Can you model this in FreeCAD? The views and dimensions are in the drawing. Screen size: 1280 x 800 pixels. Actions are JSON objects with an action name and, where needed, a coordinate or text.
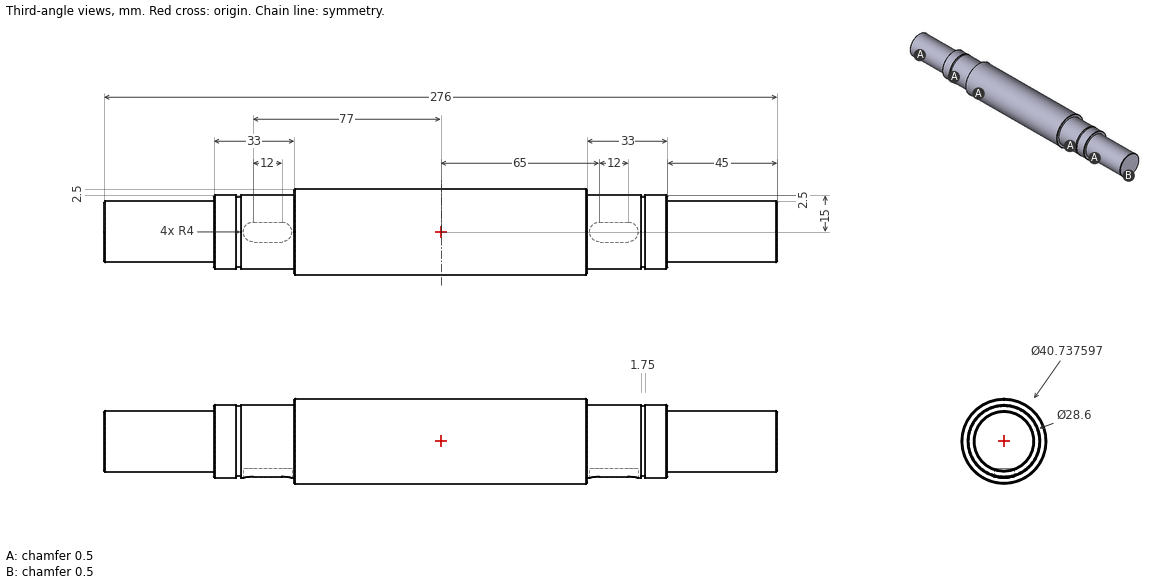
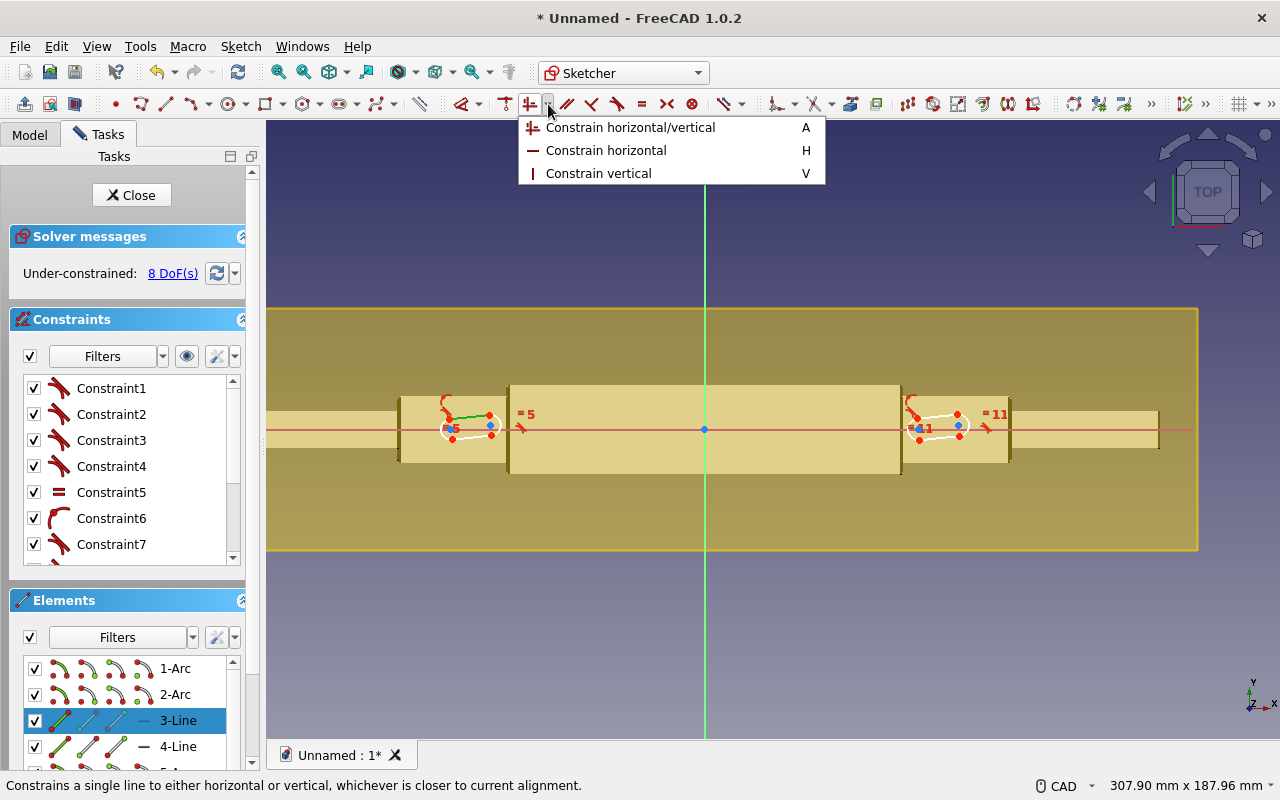
{"action": "left_click", "coordinate": [672, 150]}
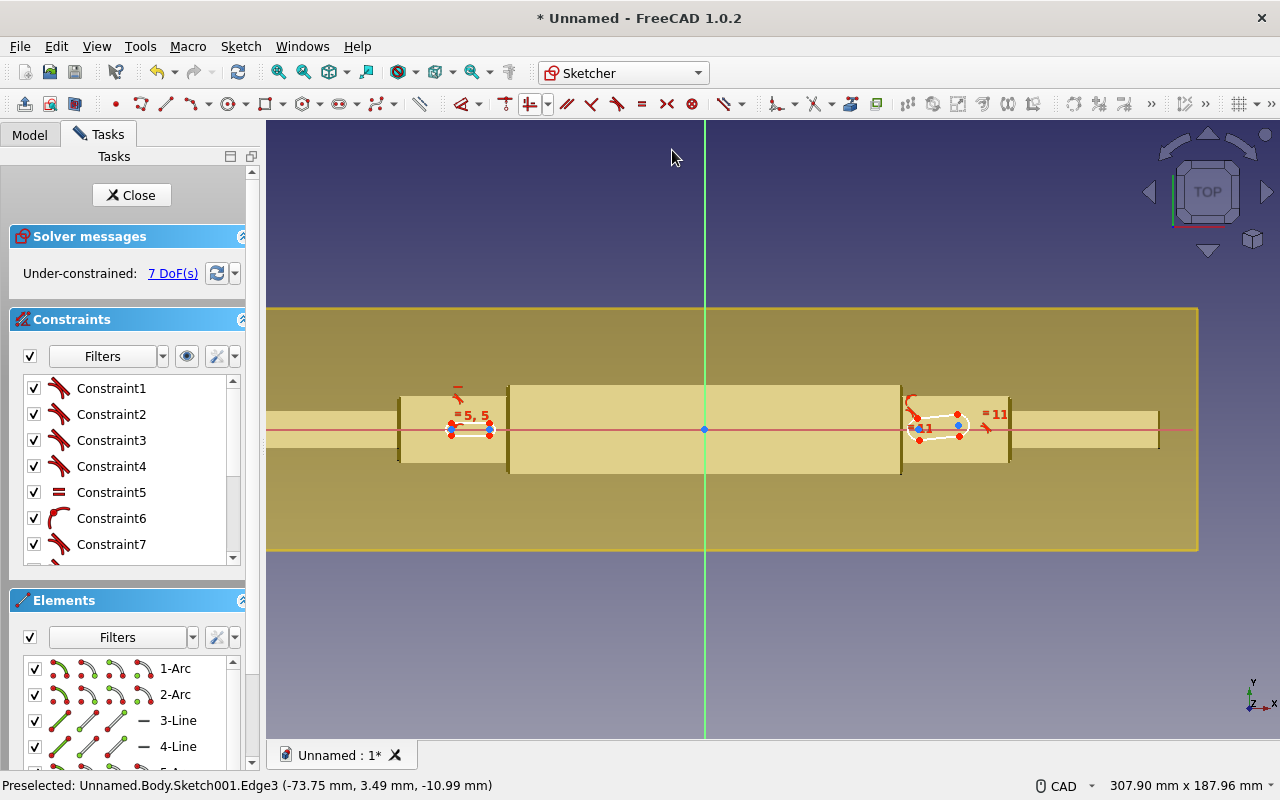
{"action": "left_click", "coordinate": [945, 416]}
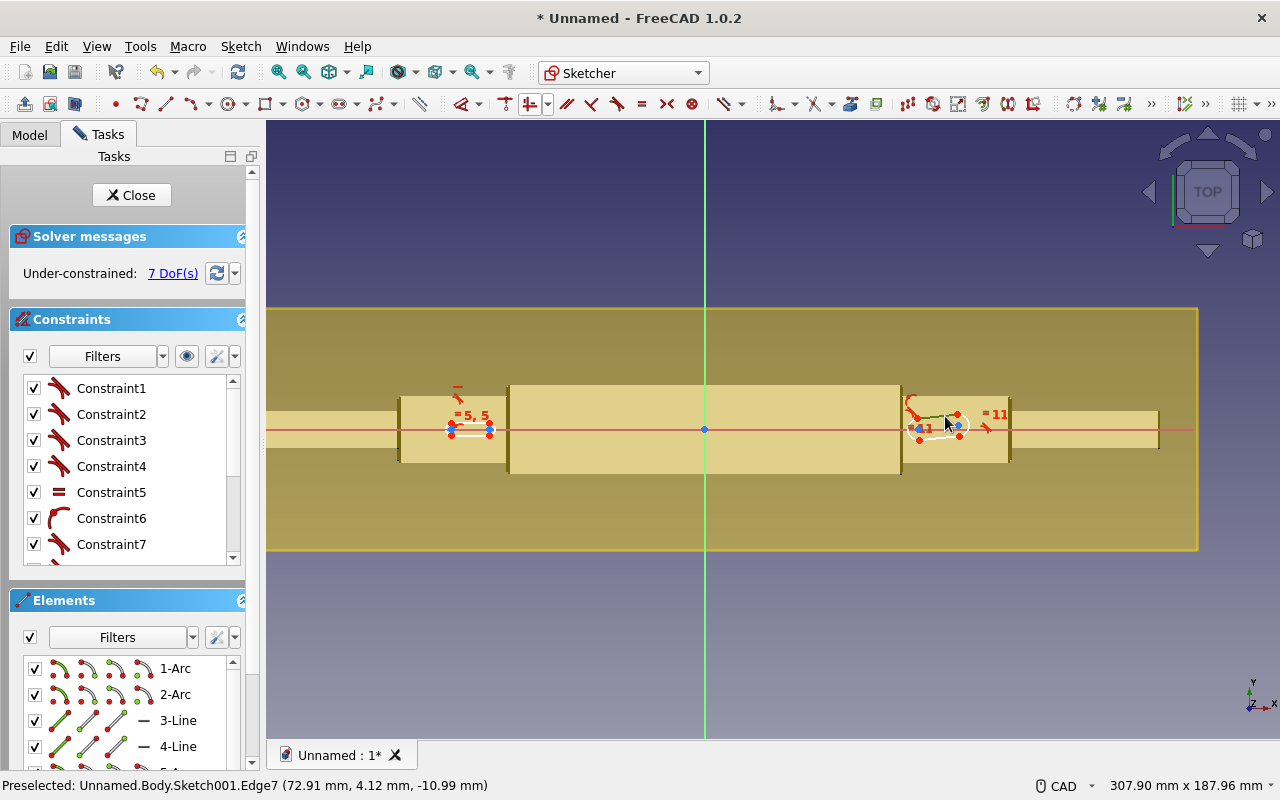
{"action": "key", "text": "h"}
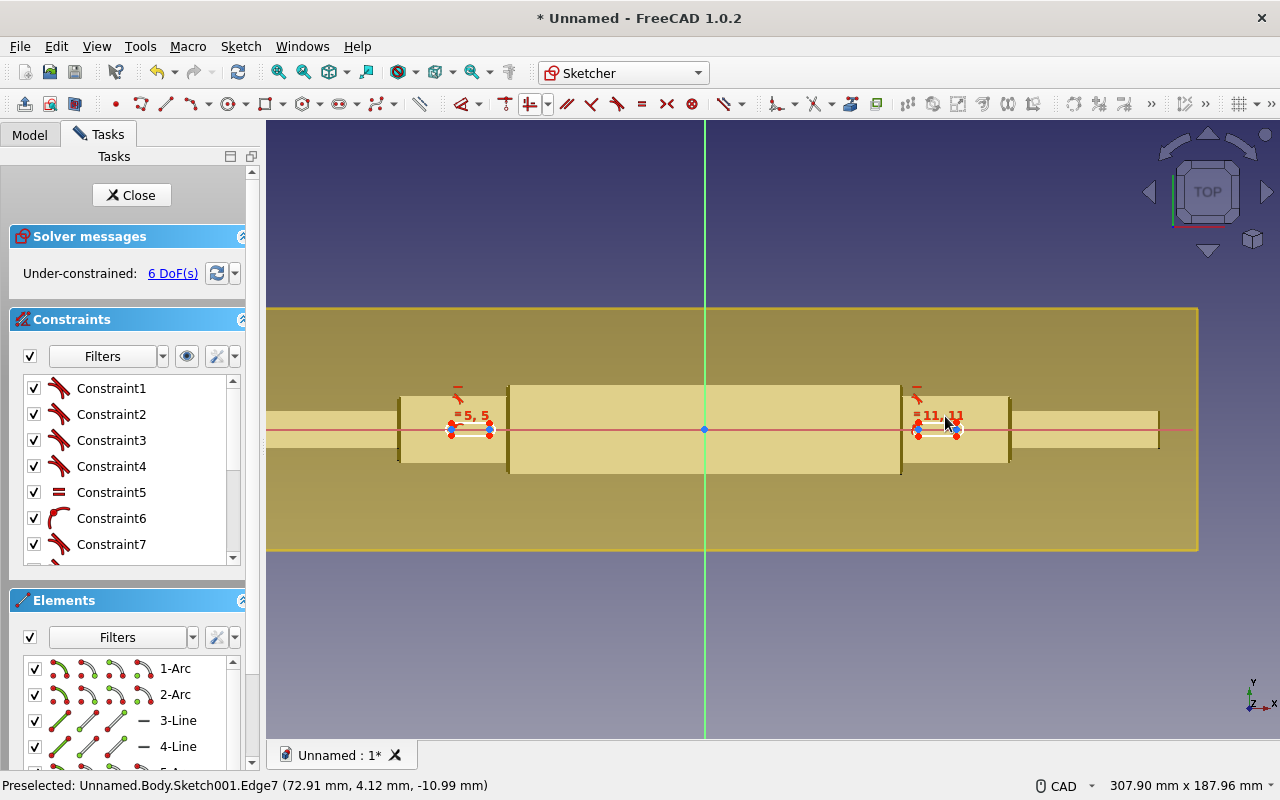
{"action": "scroll", "coordinate": [446, 430], "scroll_direction": "up", "scroll_amount": 5}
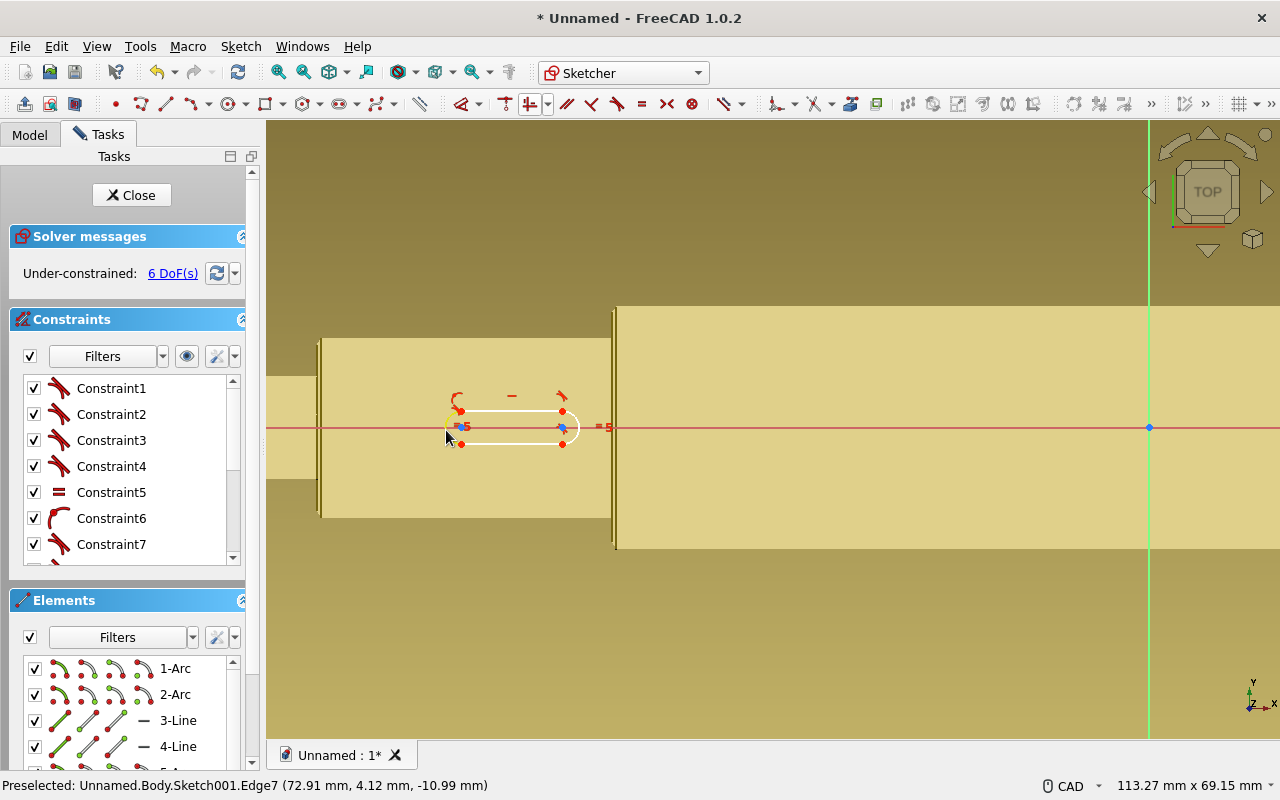
{"action": "left_click", "coordinate": [446, 428]}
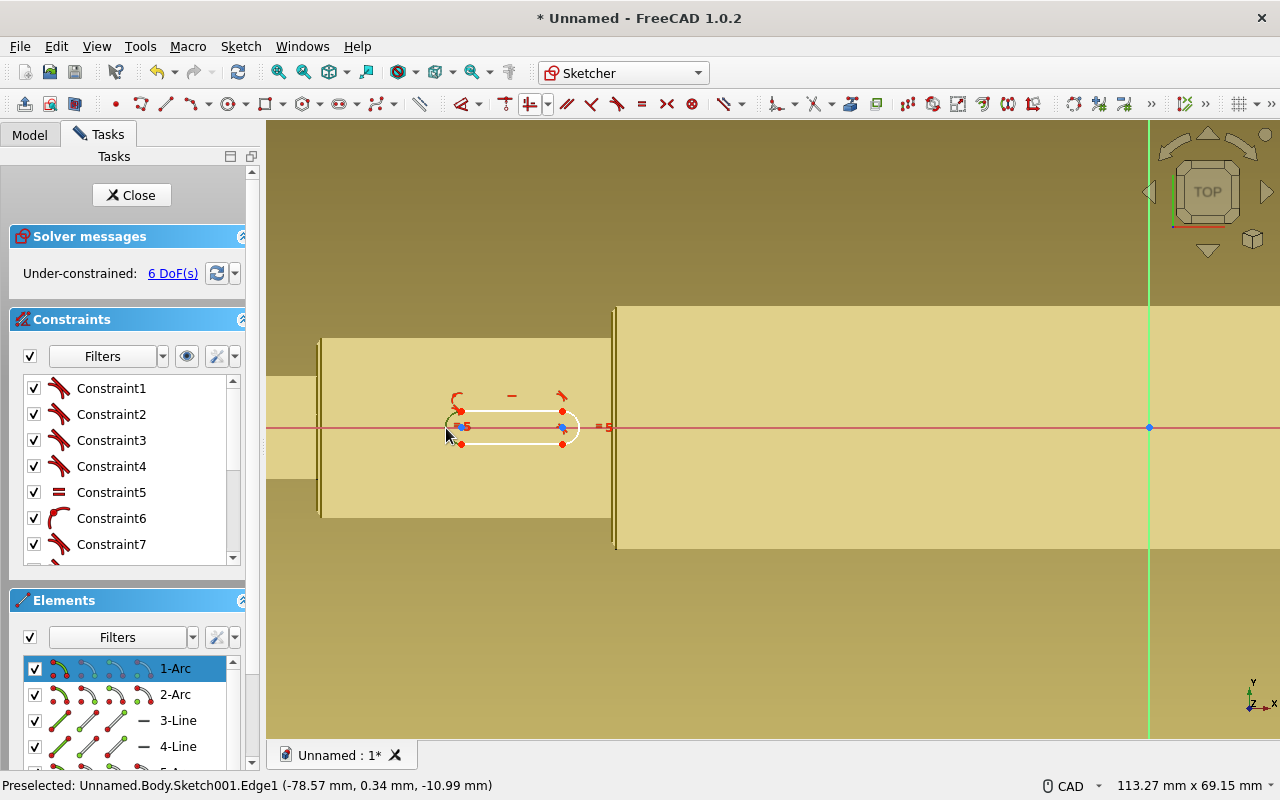
{"action": "scroll", "coordinate": [446, 431], "scroll_direction": "down", "scroll_amount": 5}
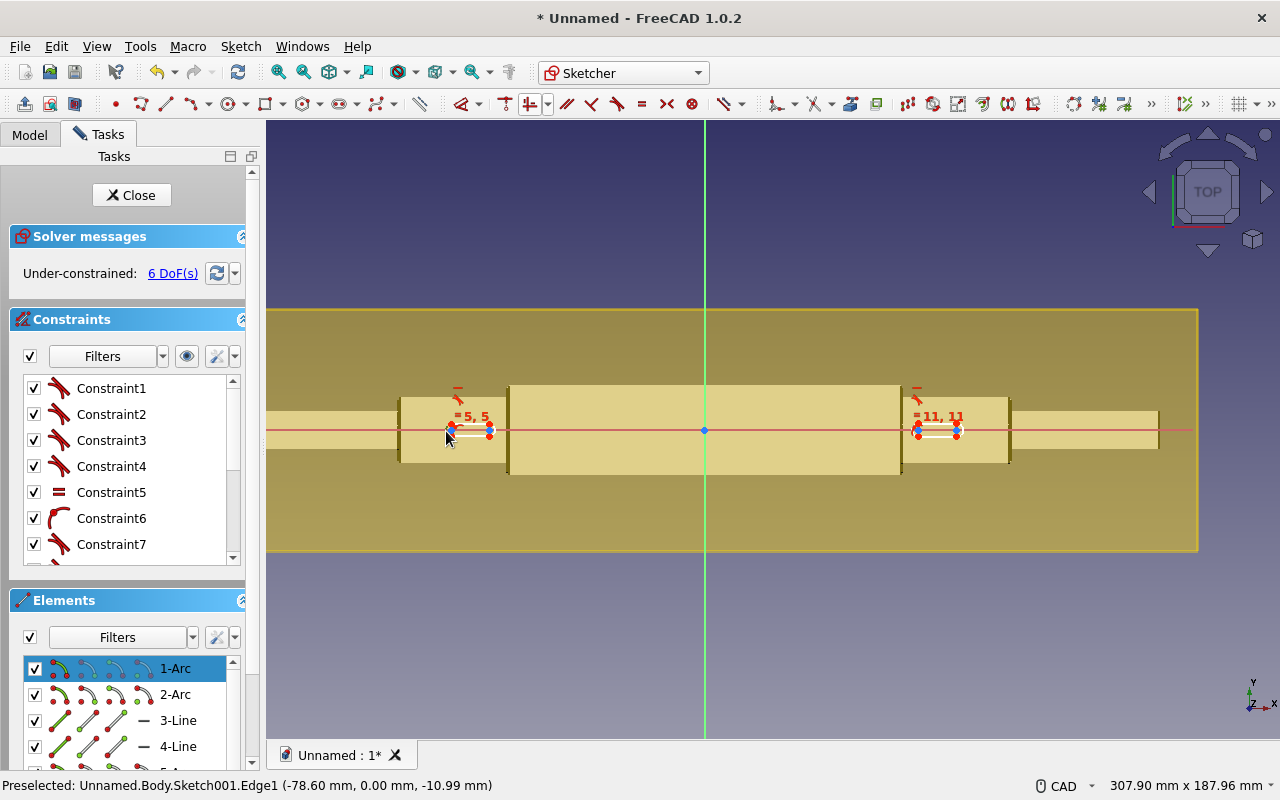
{"action": "scroll", "coordinate": [914, 426], "scroll_direction": "up", "scroll_amount": 7}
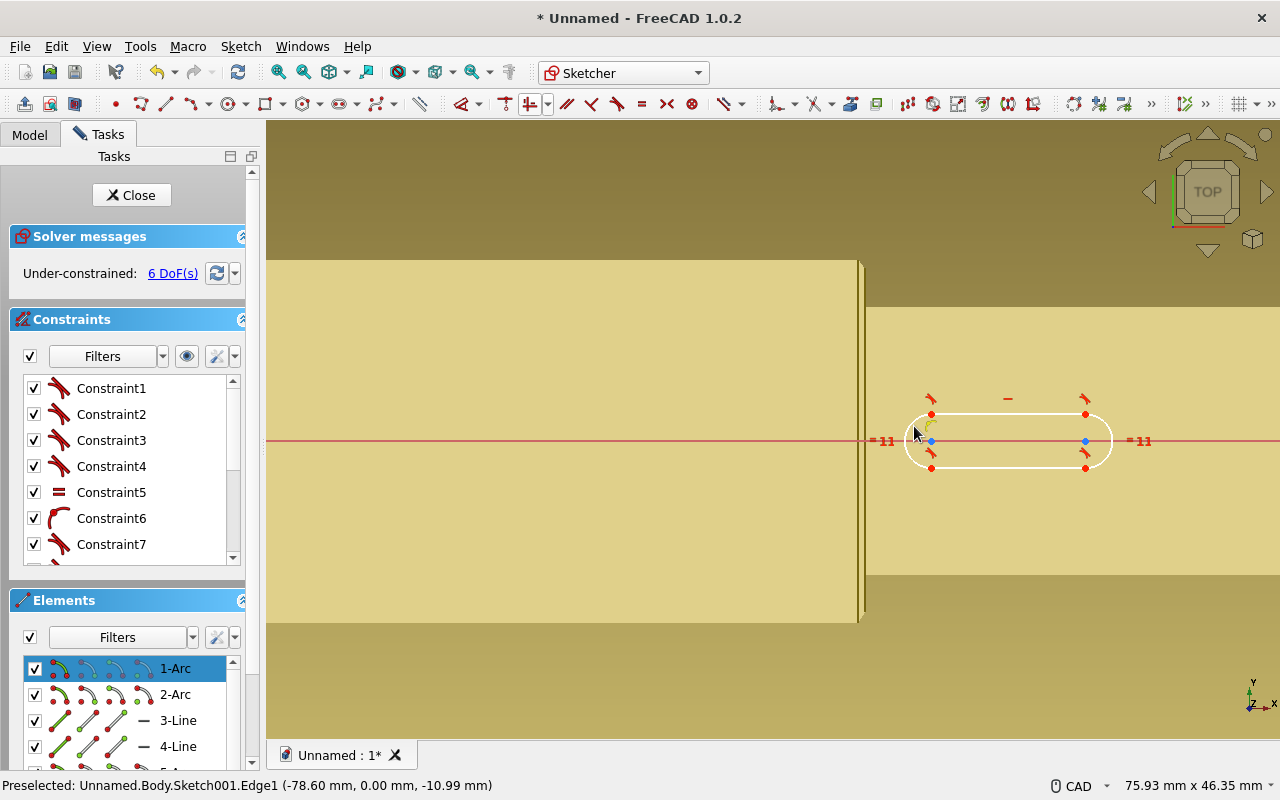
{"action": "left_click", "coordinate": [910, 425]}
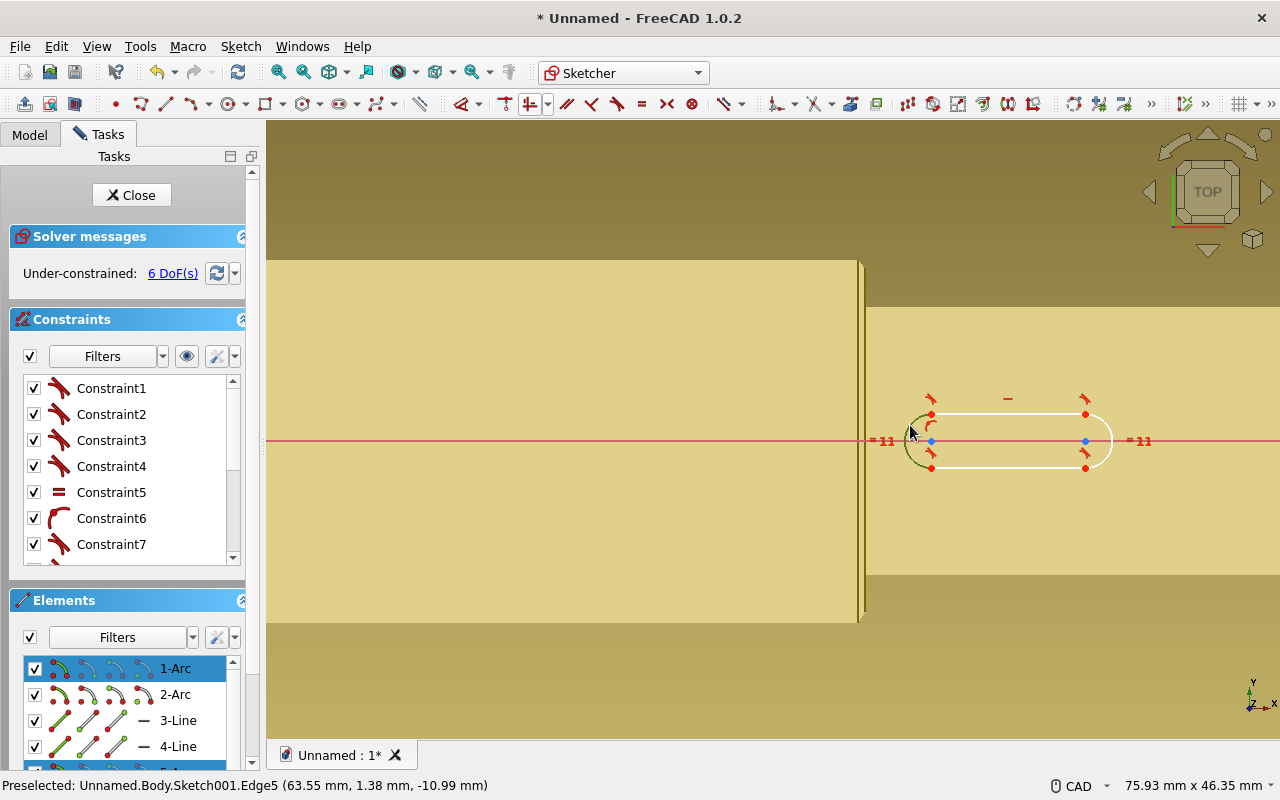
{"action": "left_click", "coordinate": [642, 104]}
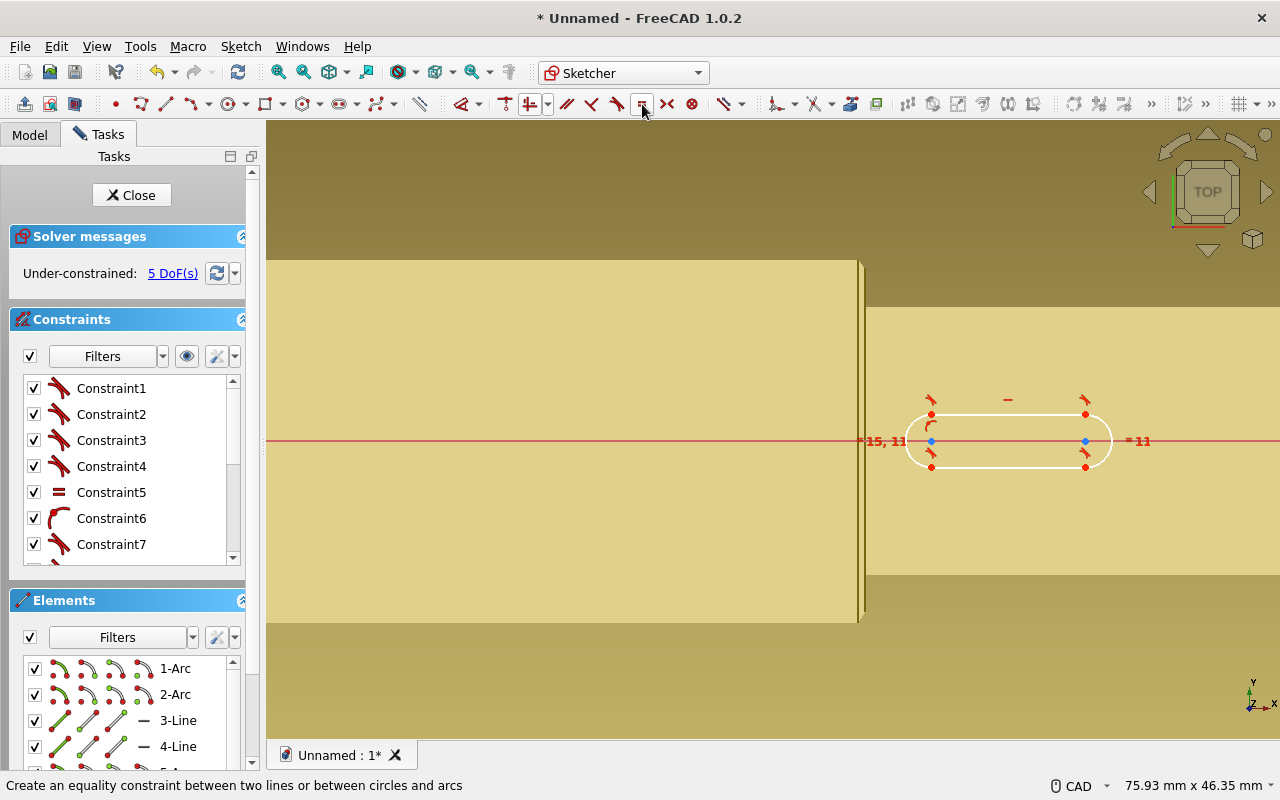
{"action": "left_click", "coordinate": [460, 104]}